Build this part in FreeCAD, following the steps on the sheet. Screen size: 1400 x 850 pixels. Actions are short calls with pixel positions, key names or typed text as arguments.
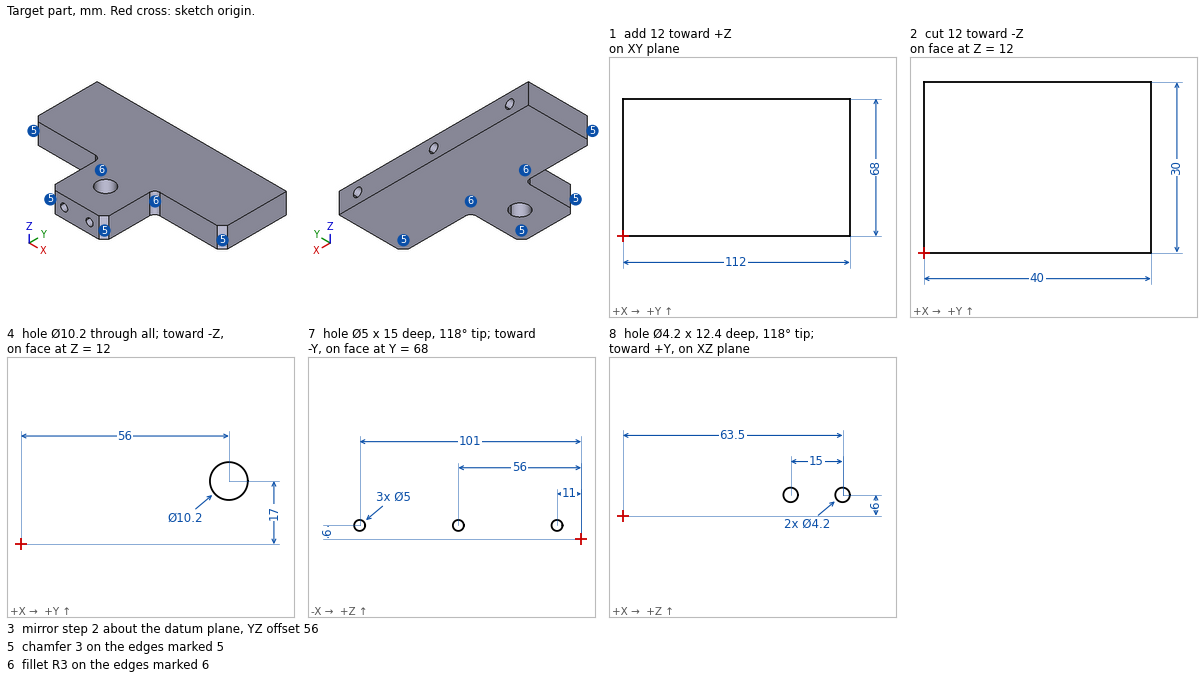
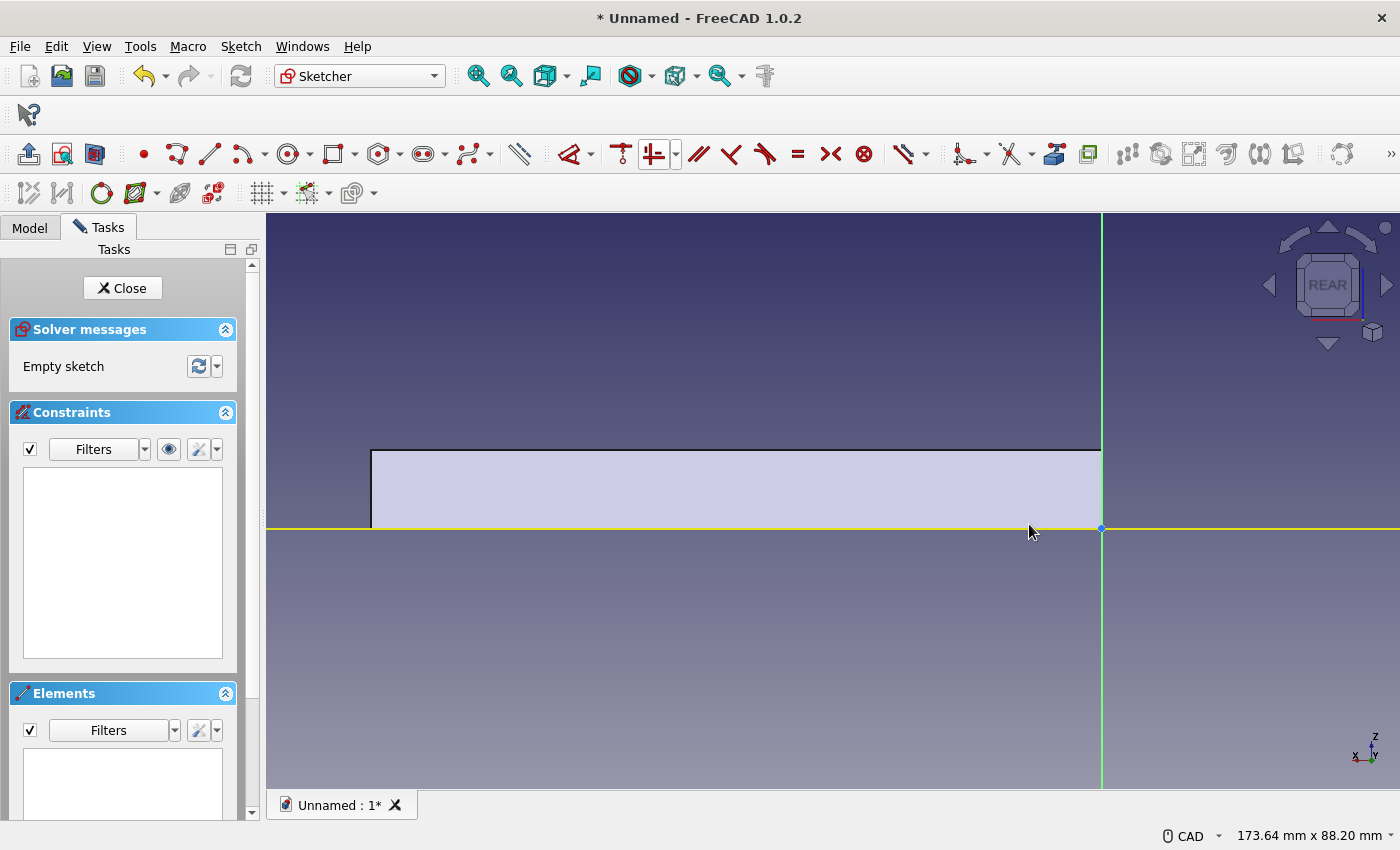
click(288, 154)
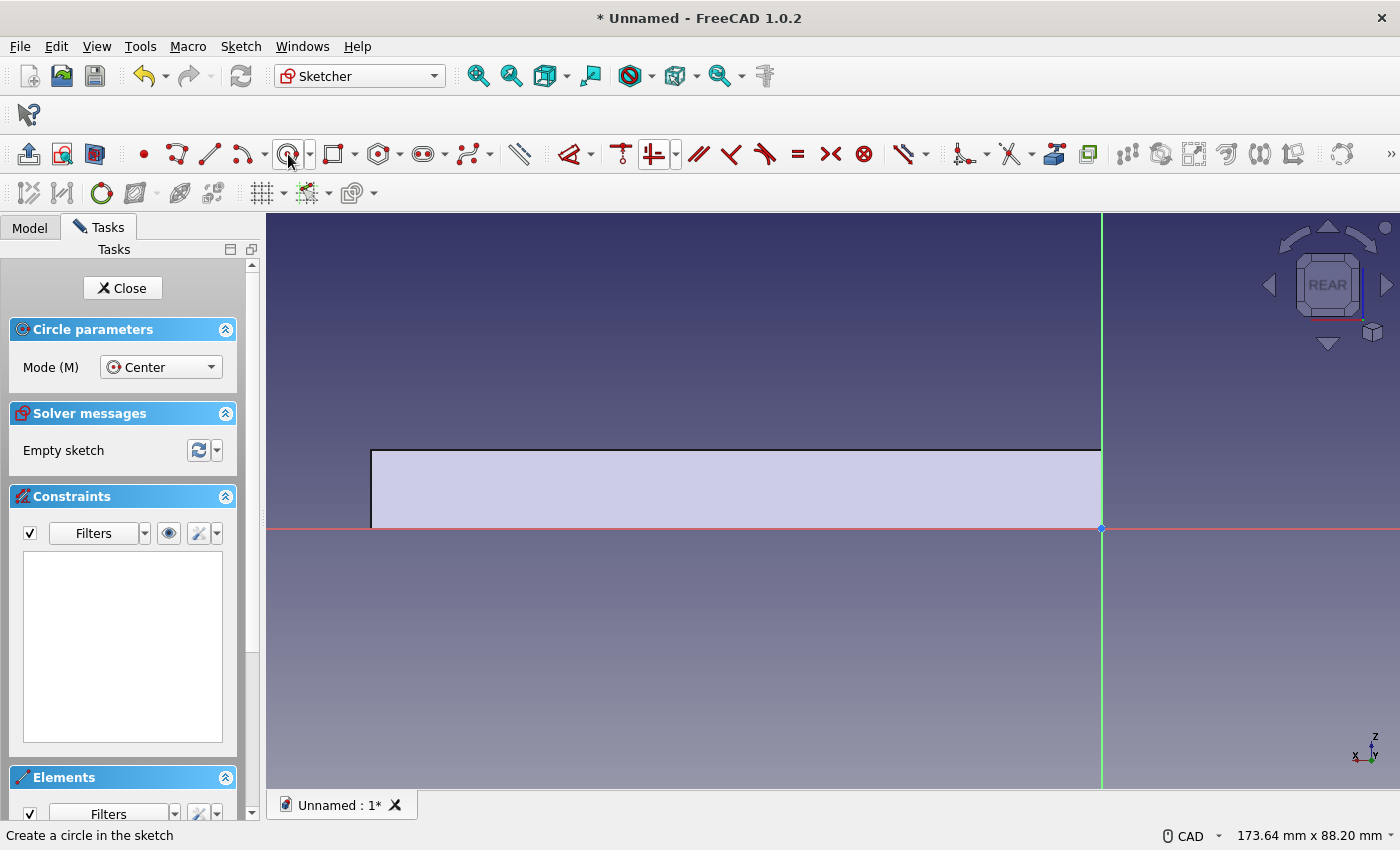
scroll(442, 489, up, 2)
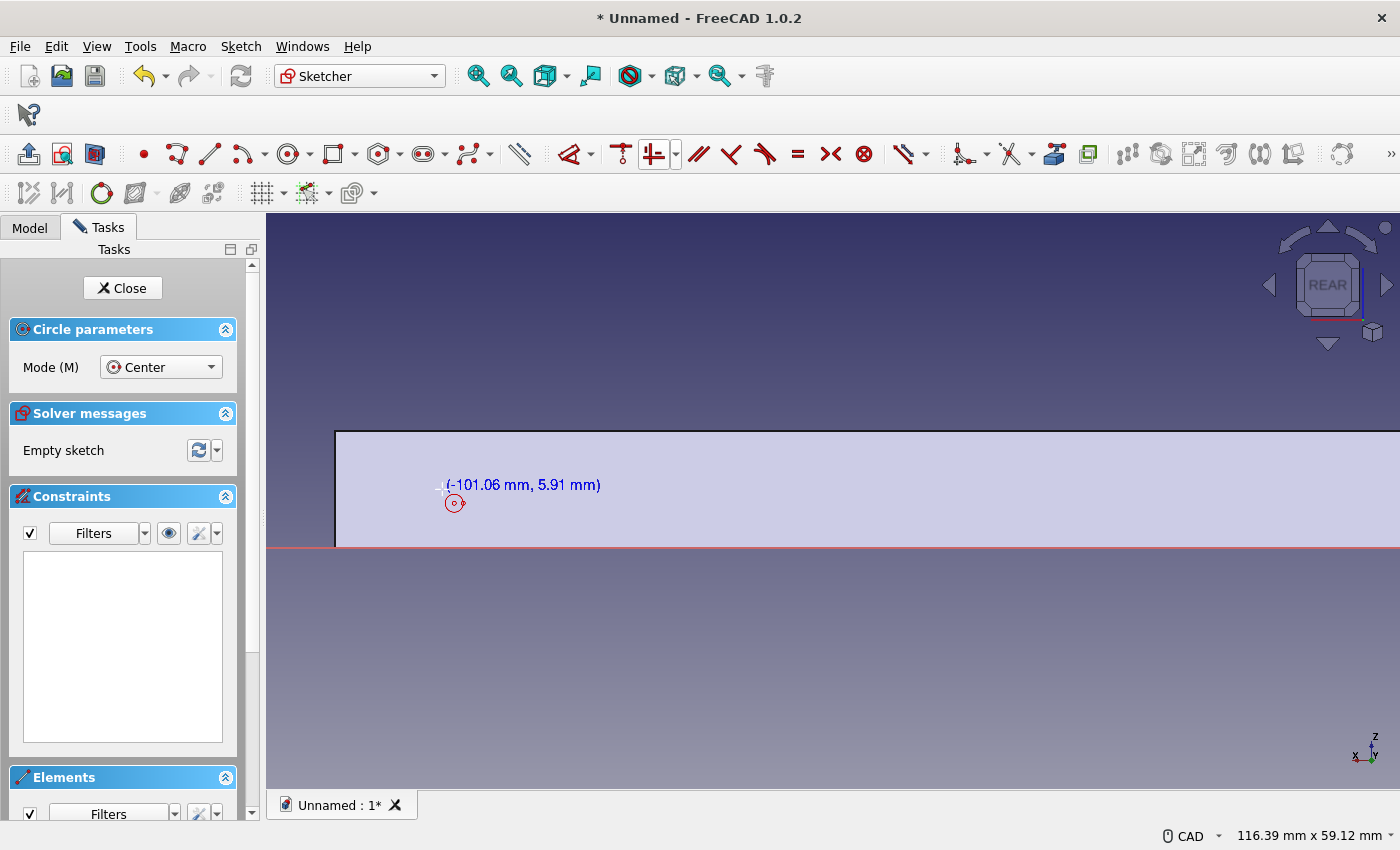
click(442, 489)
click(460, 472)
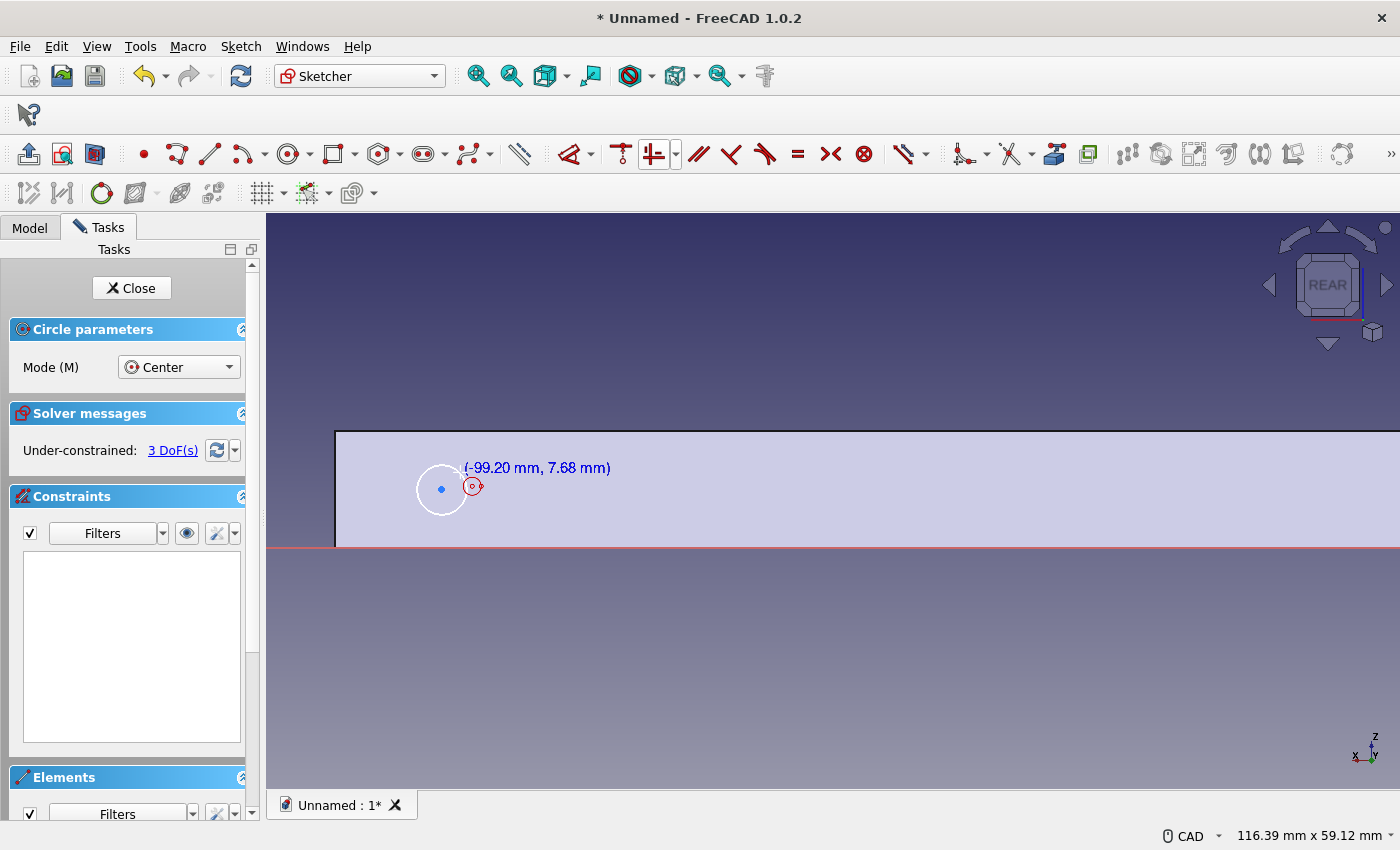
click(881, 489)
click(898, 472)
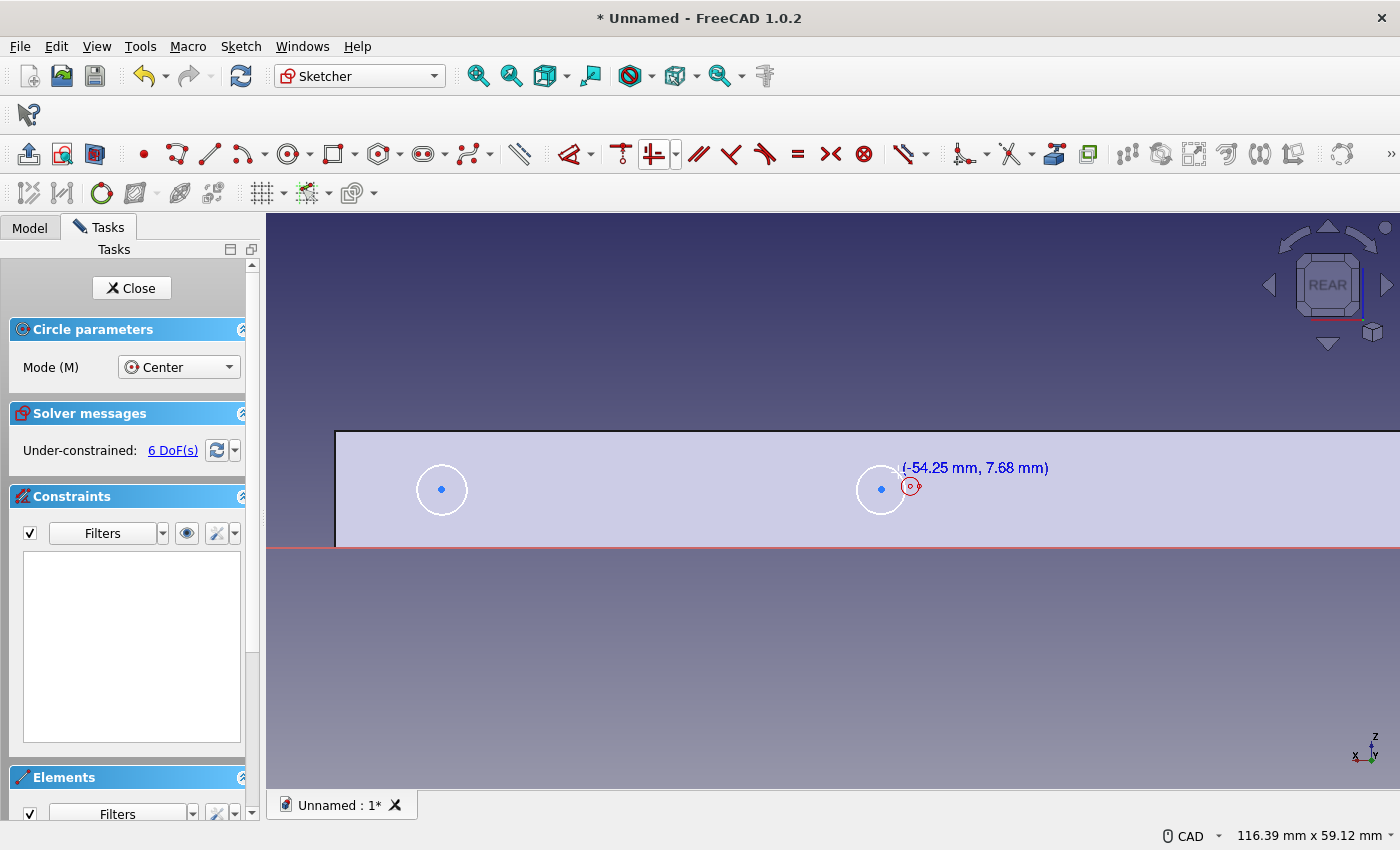
scroll(444, 490, down, 2)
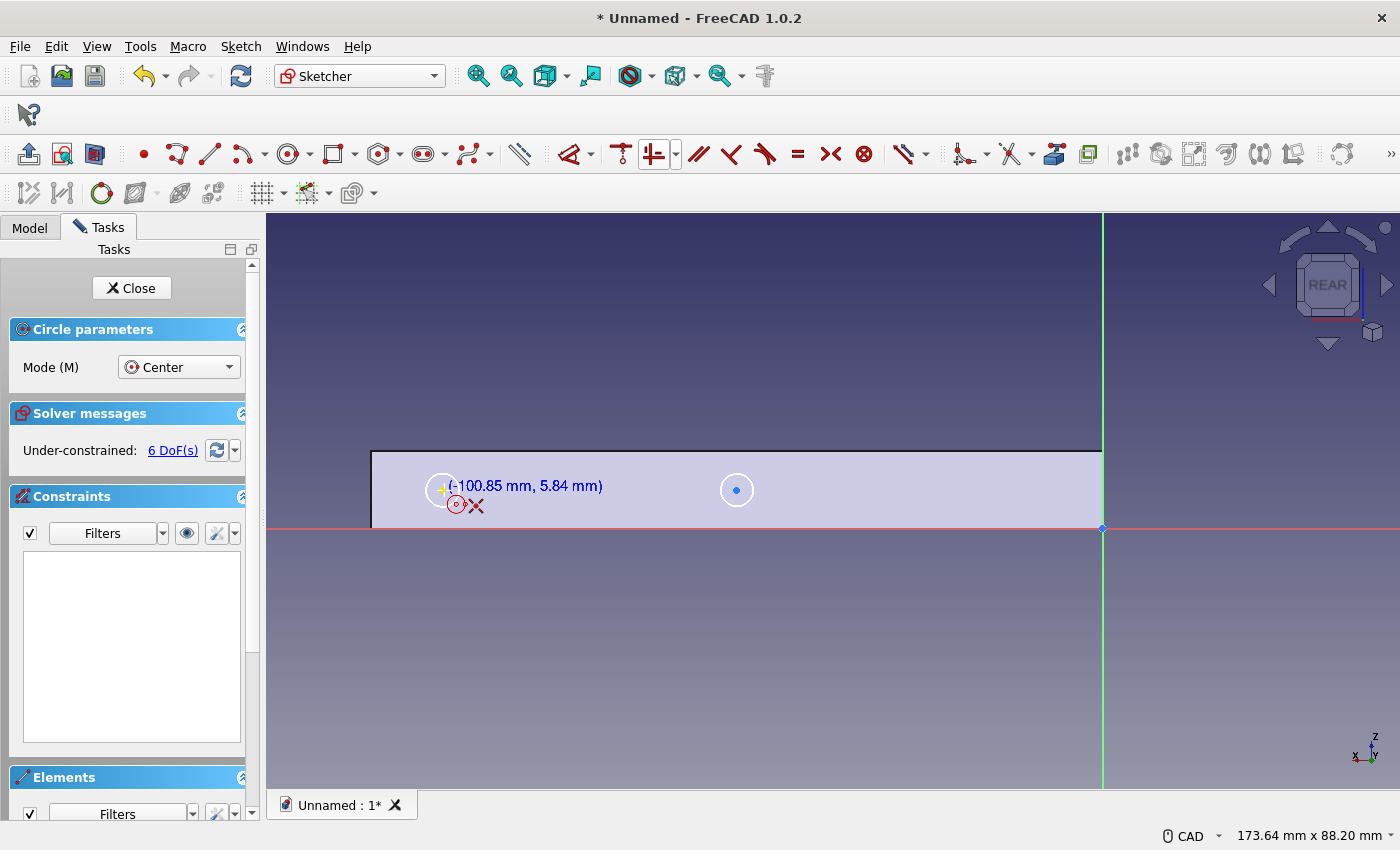
scroll(1031, 490, up, 2)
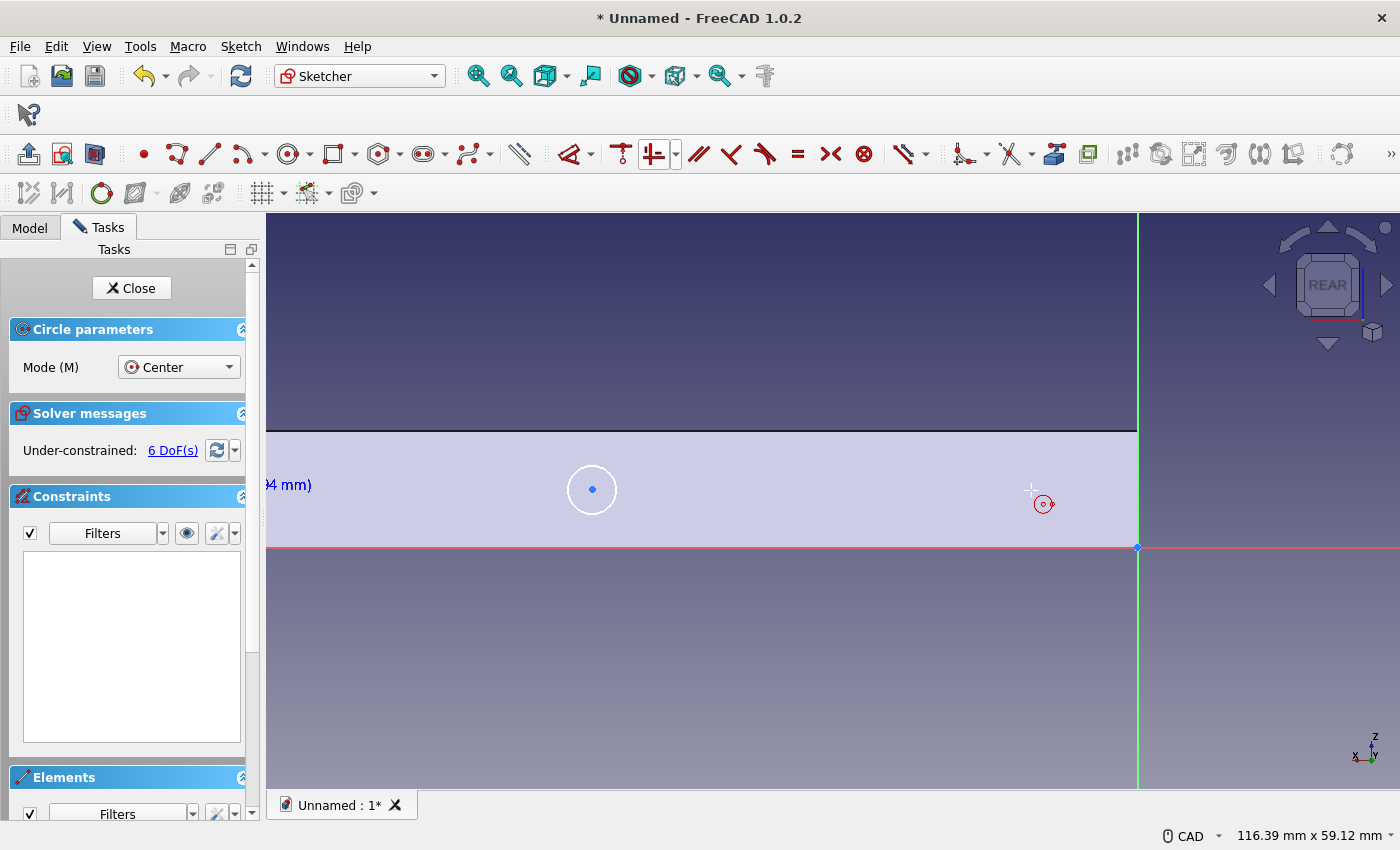
click(1030, 489)
click(1048, 472)
key(Escape)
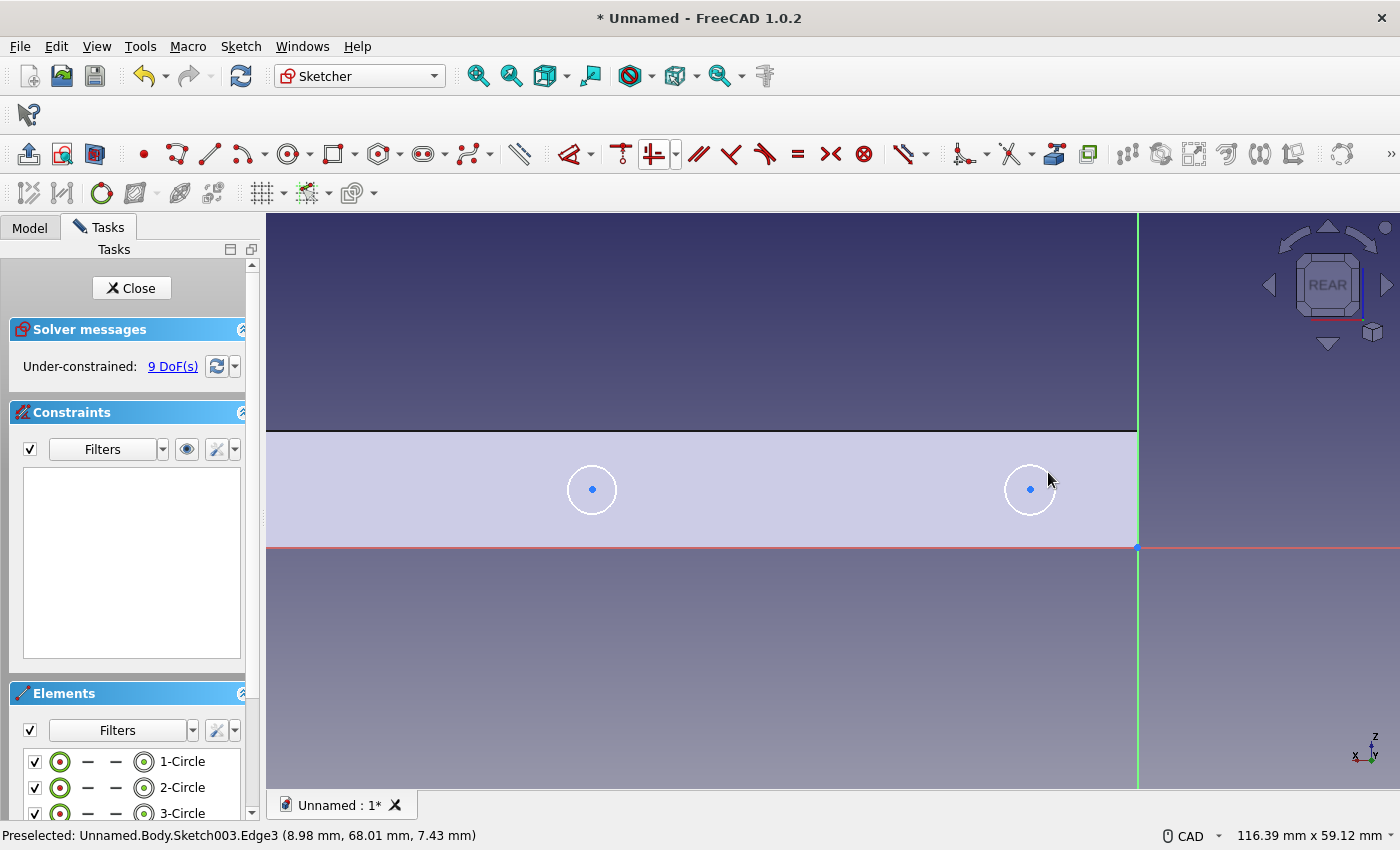
scroll(1031, 490, down, 2)